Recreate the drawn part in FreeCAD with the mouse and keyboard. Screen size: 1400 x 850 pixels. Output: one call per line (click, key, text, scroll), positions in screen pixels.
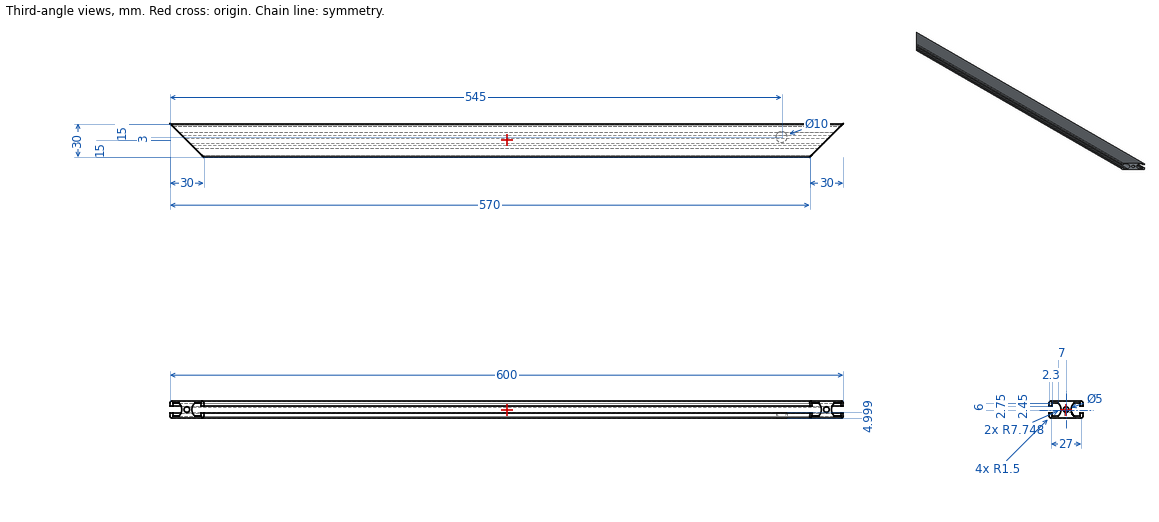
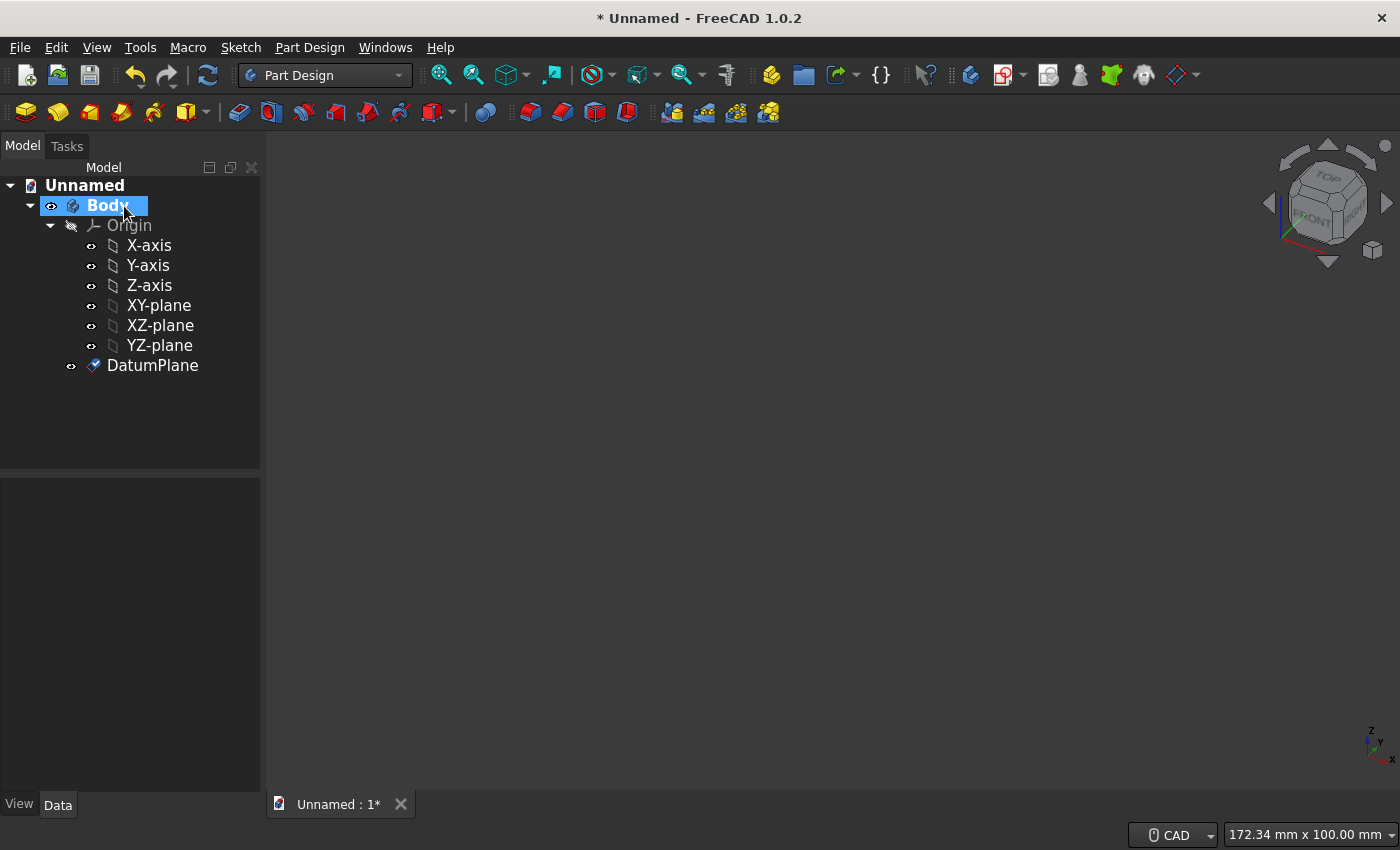
click(116, 366)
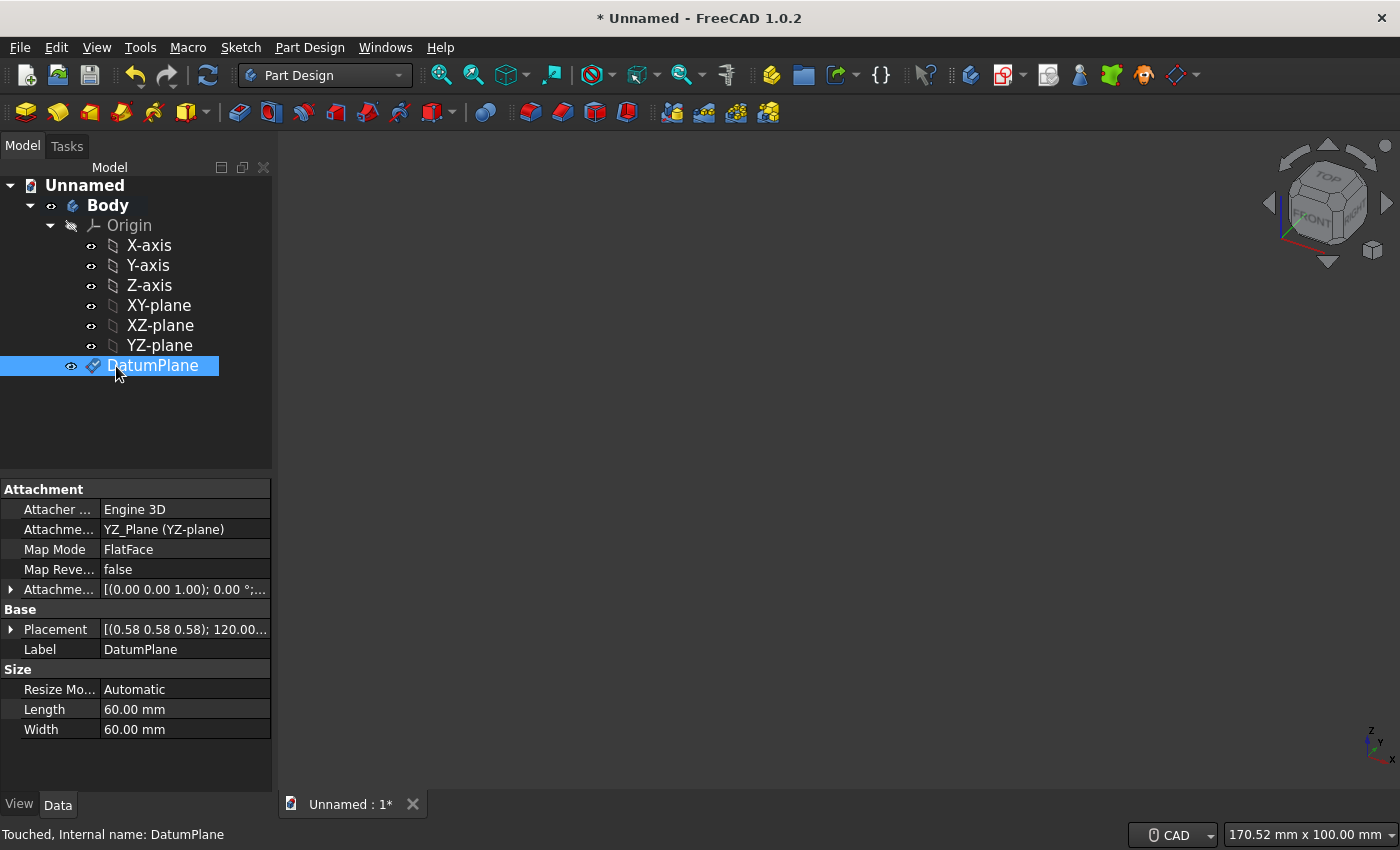
click(1004, 76)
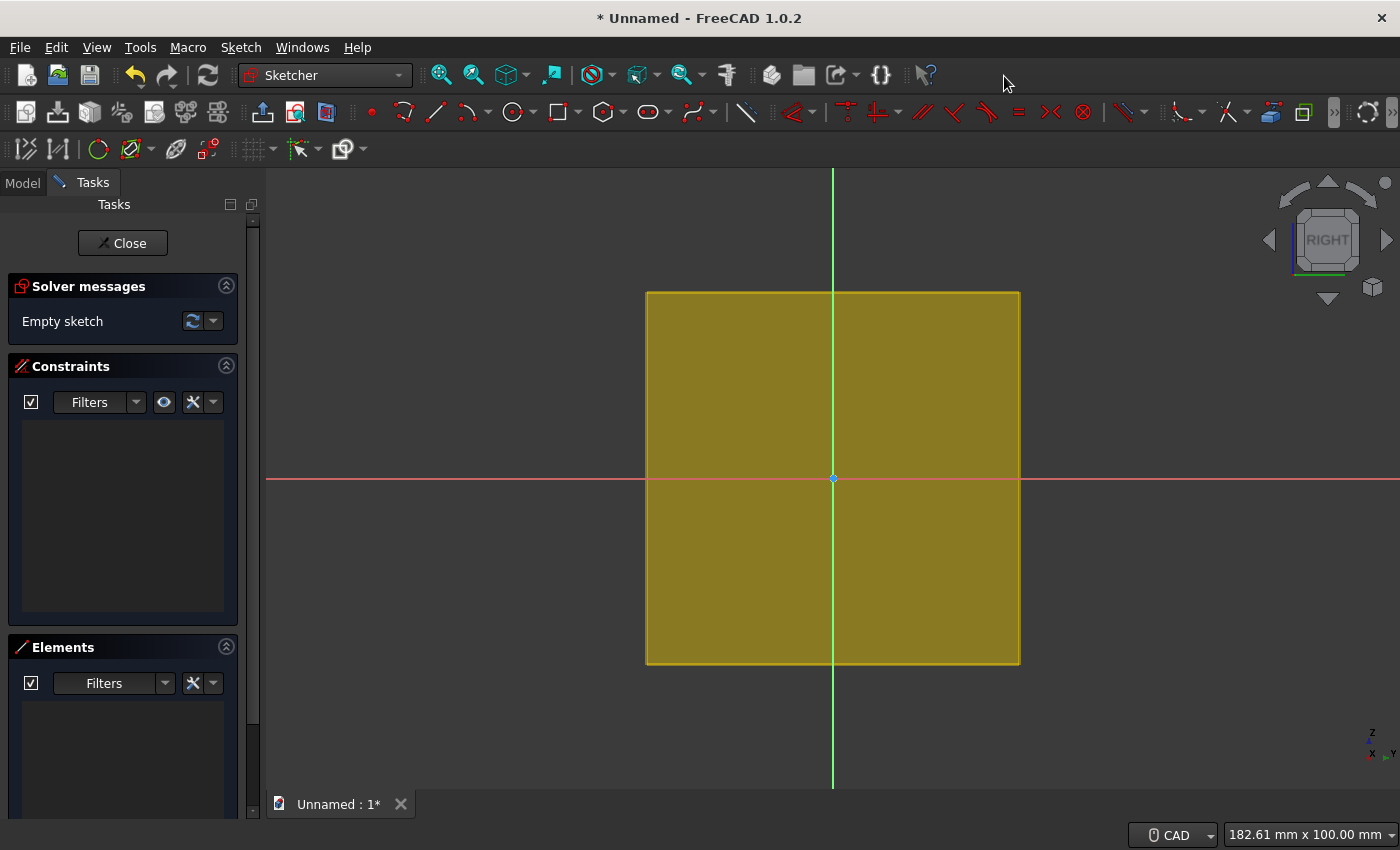
scroll(863, 478, up, 6)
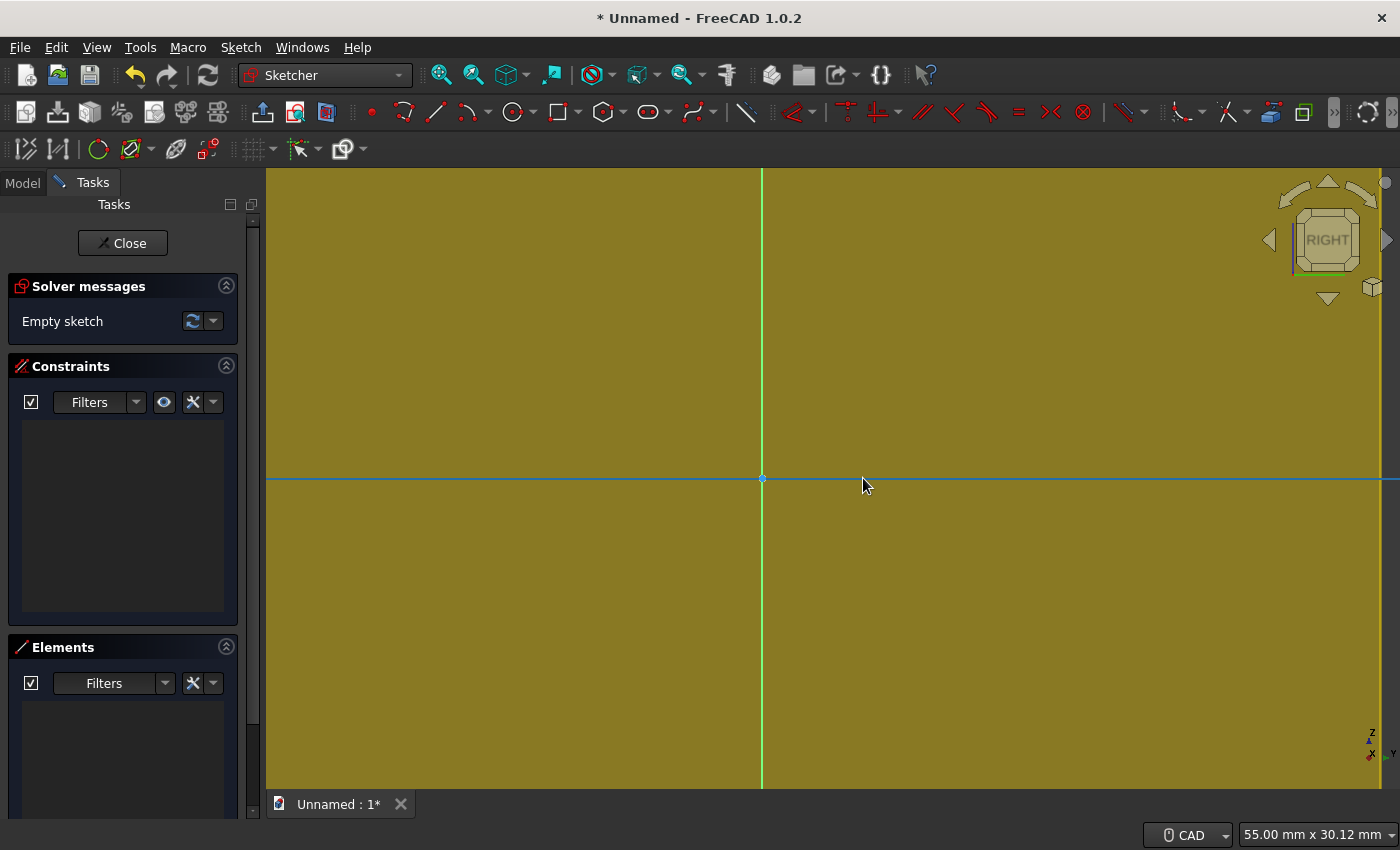
key(g)
key(m)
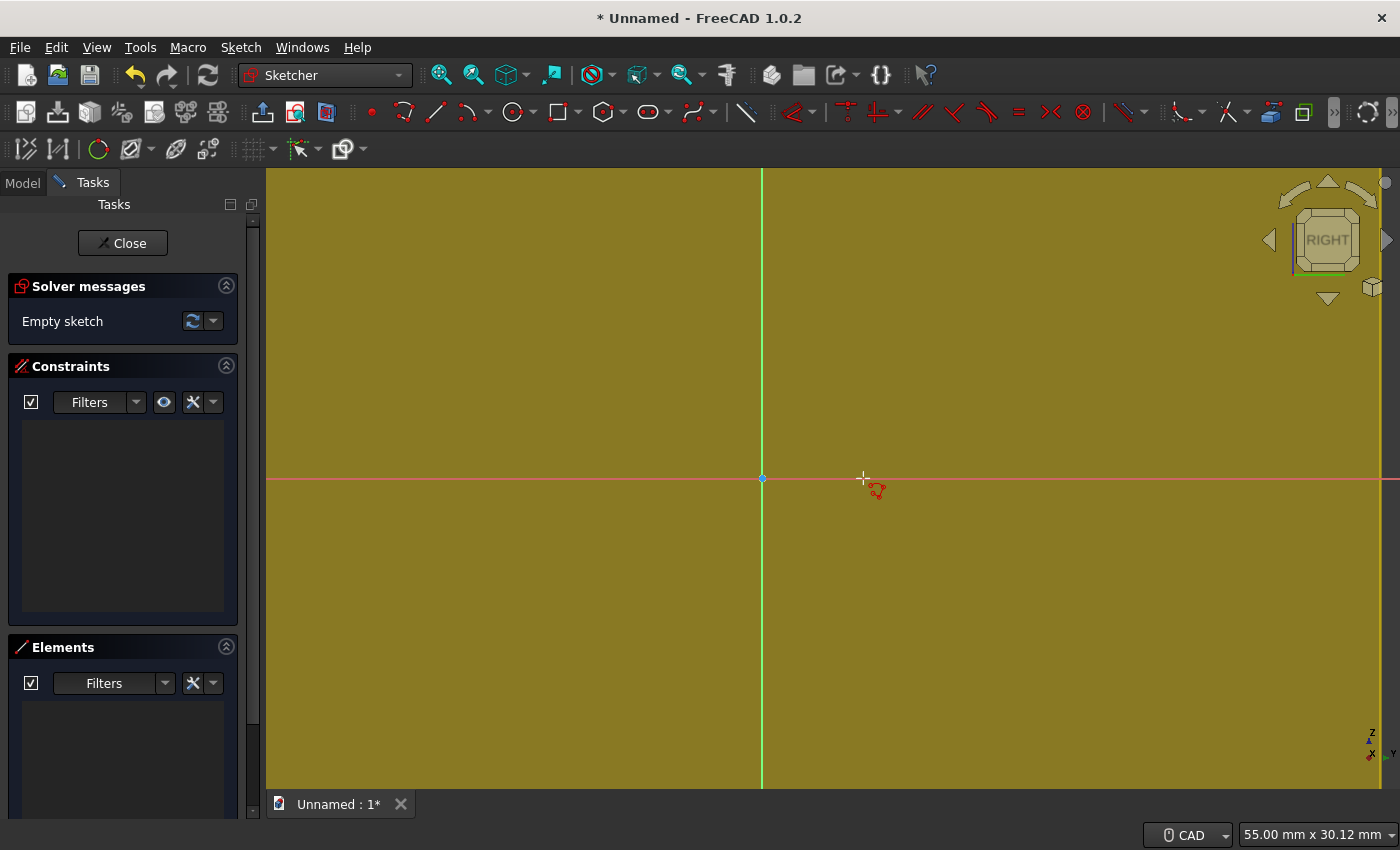
click(453, 355)
click(453, 411)
click(500, 411)
click(500, 361)
click(618, 361)
right_click(618, 361)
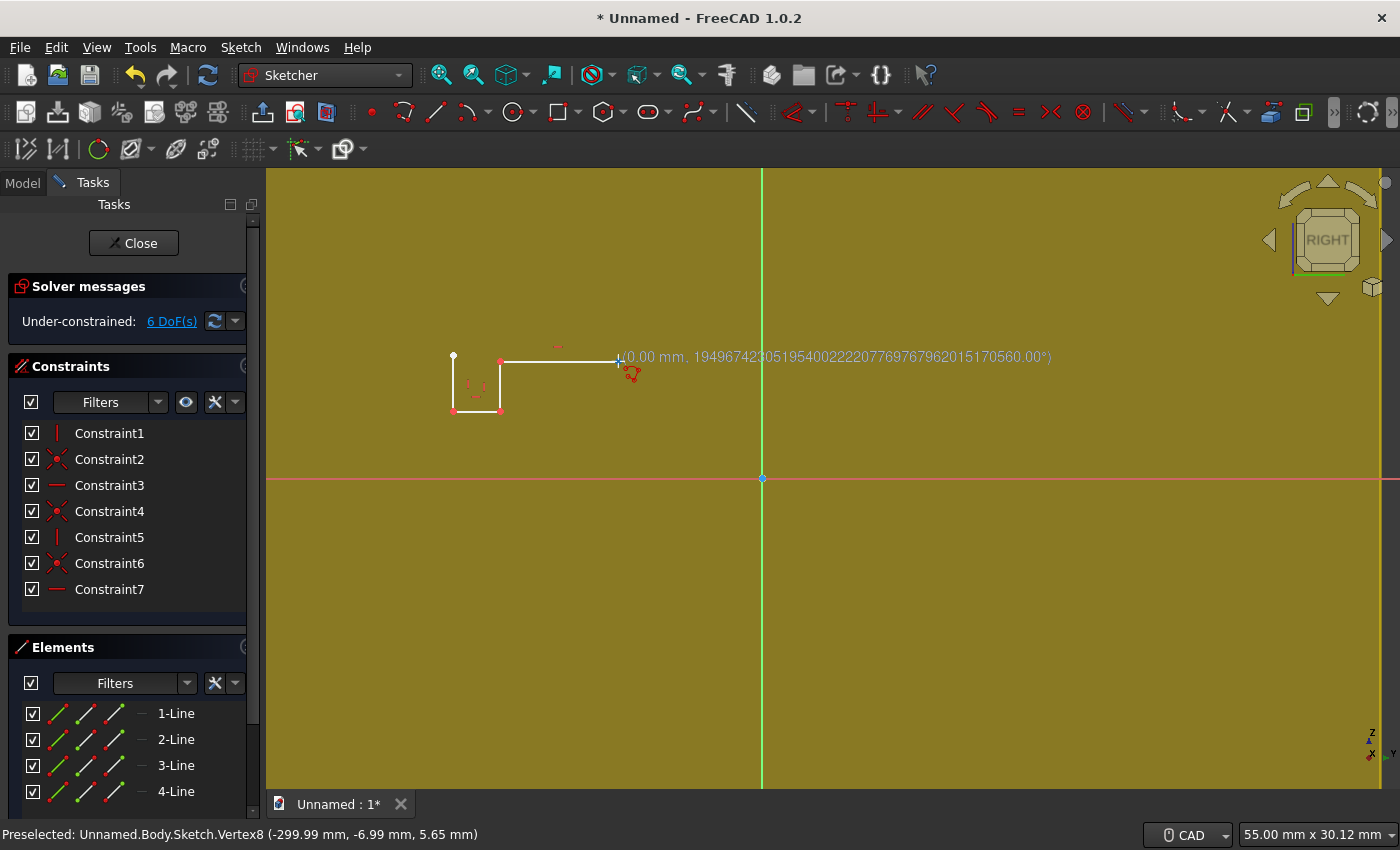
click(618, 596)
click(500, 596)
click(500, 546)
click(453, 546)
click(453, 602)
right_click(453, 602)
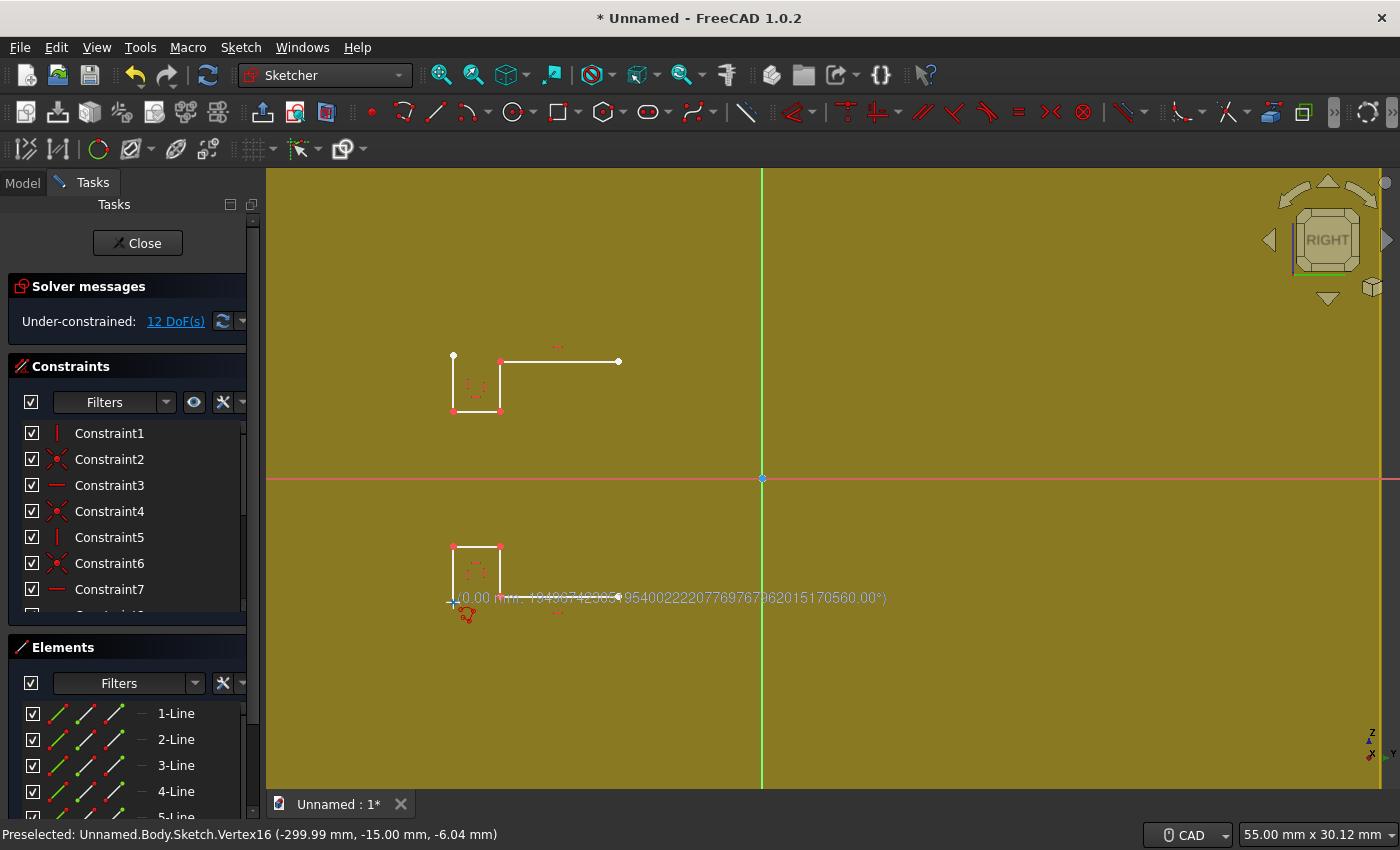
key(g)
key(l)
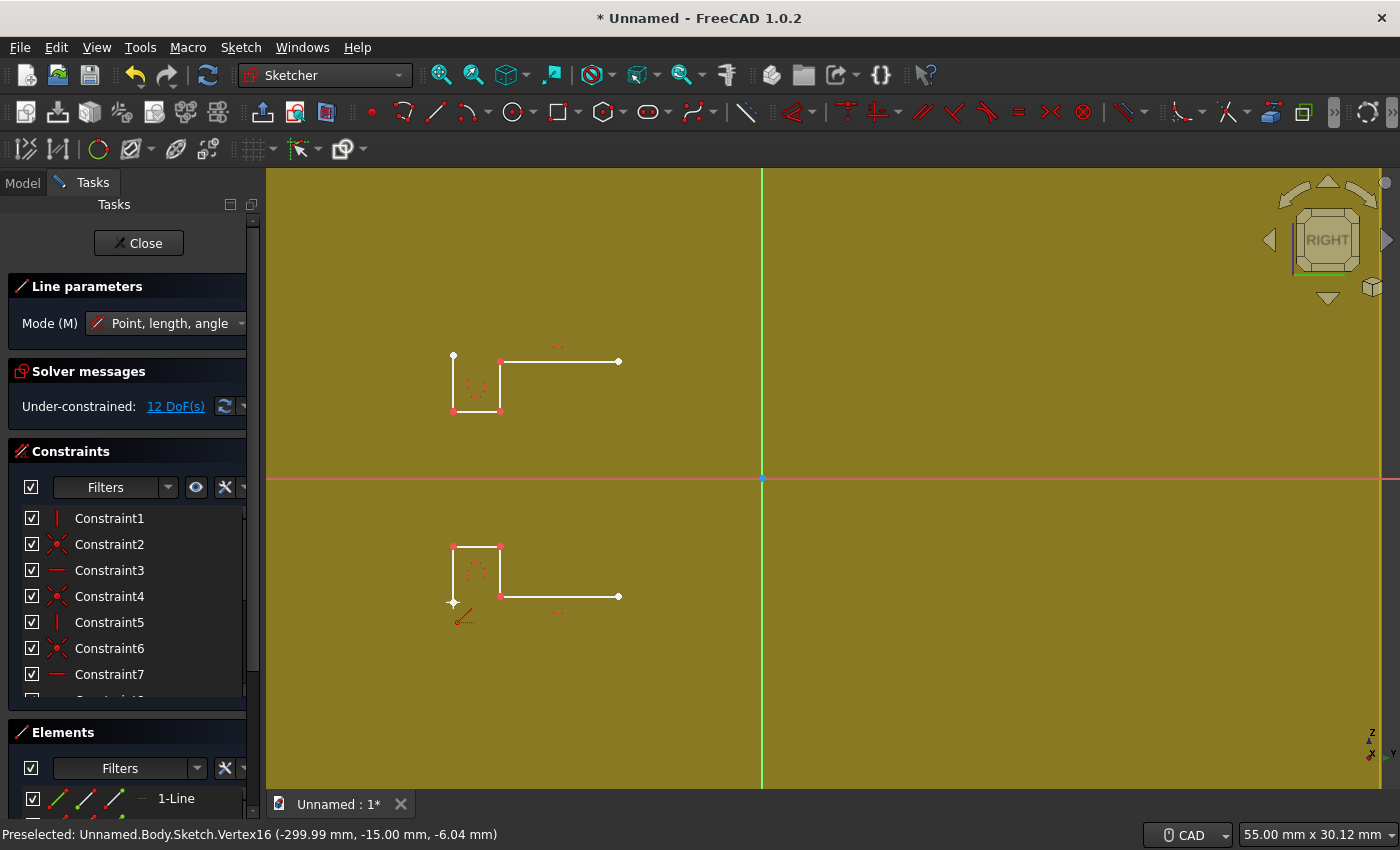
click(484, 633)
click(1041, 633)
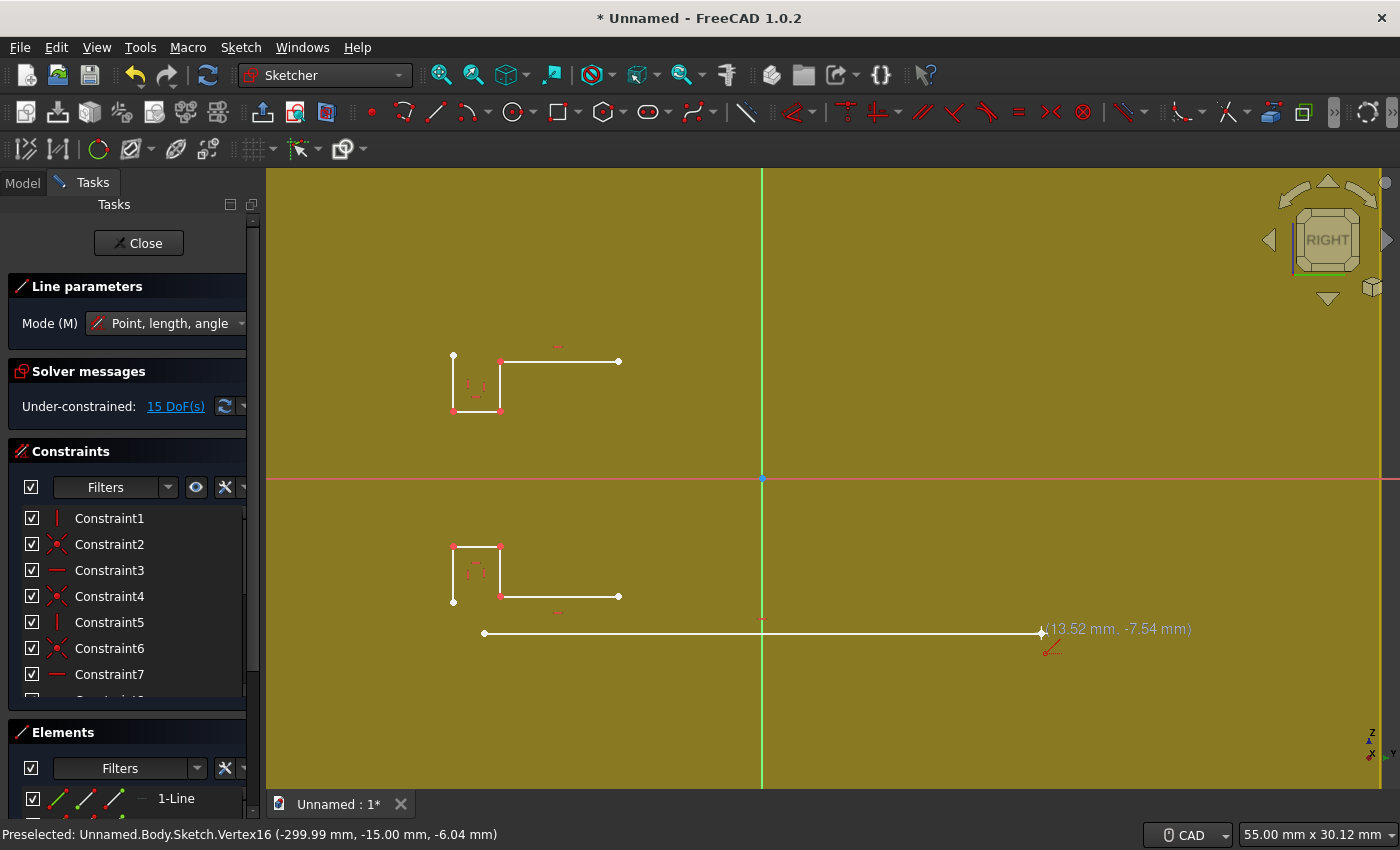
key(g)
key(m)